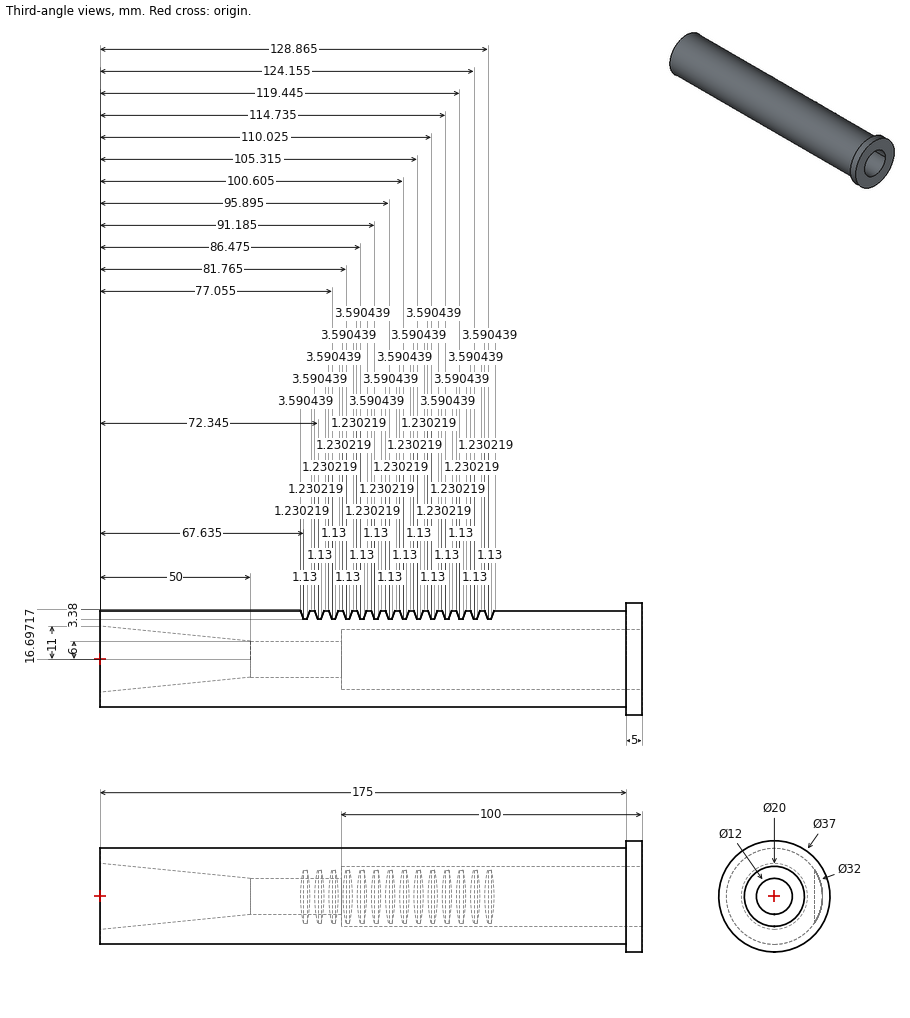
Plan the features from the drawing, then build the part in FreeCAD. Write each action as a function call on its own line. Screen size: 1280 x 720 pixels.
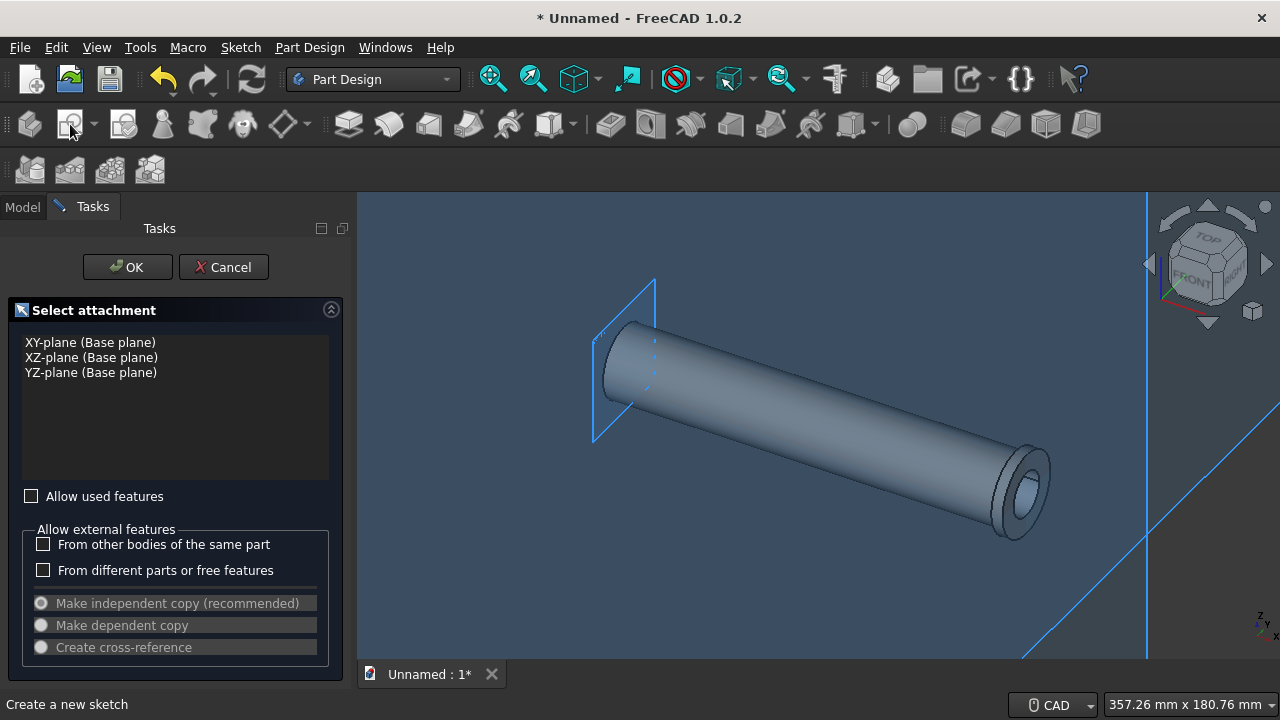
click(82, 342)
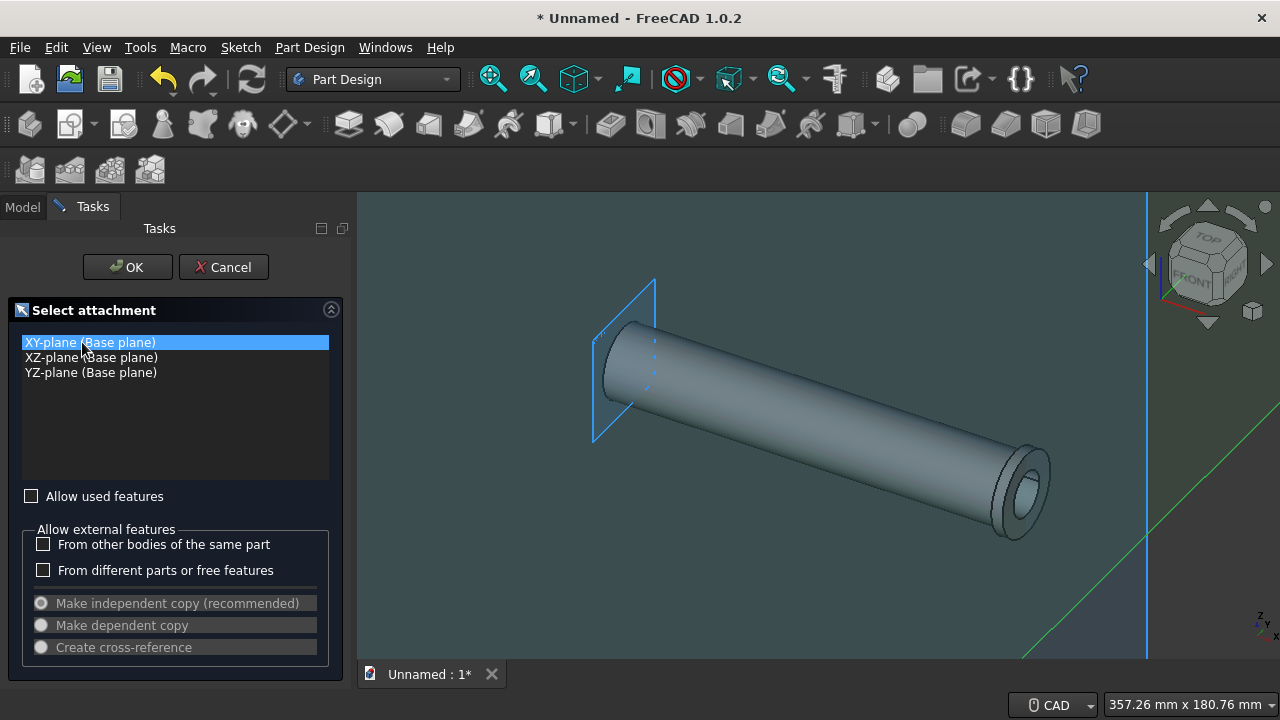
click(128, 267)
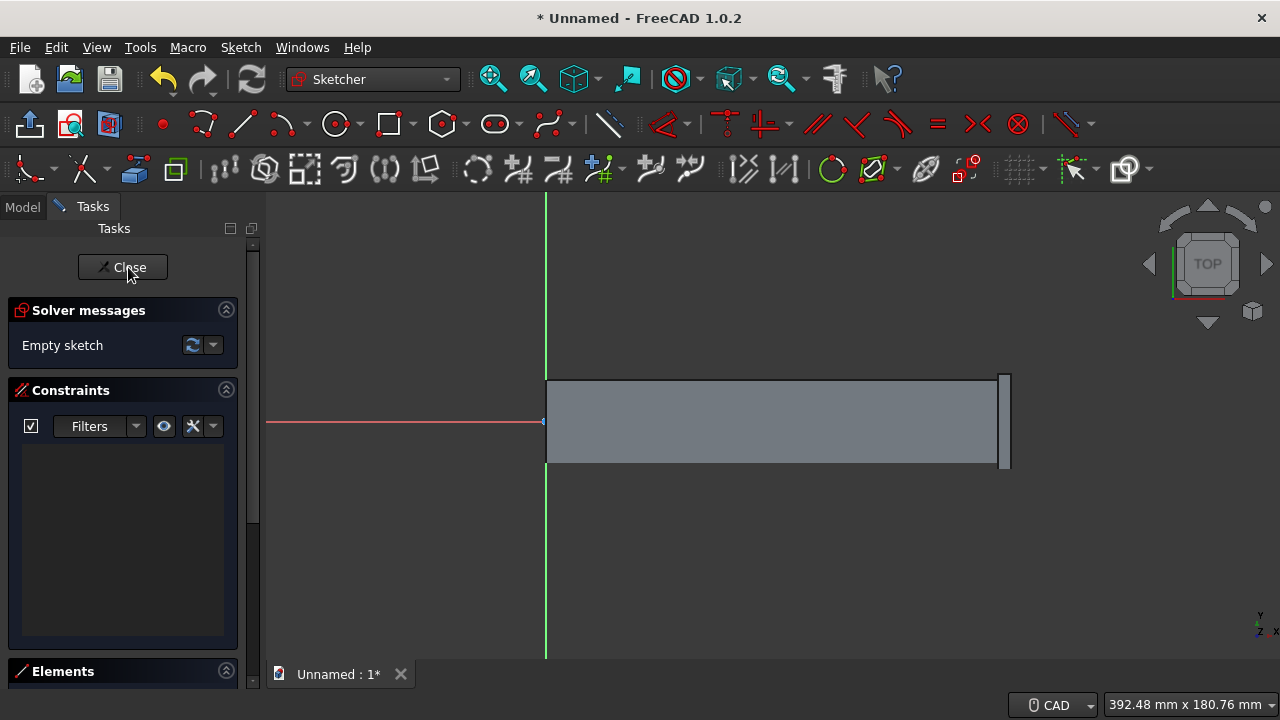
click(110, 124)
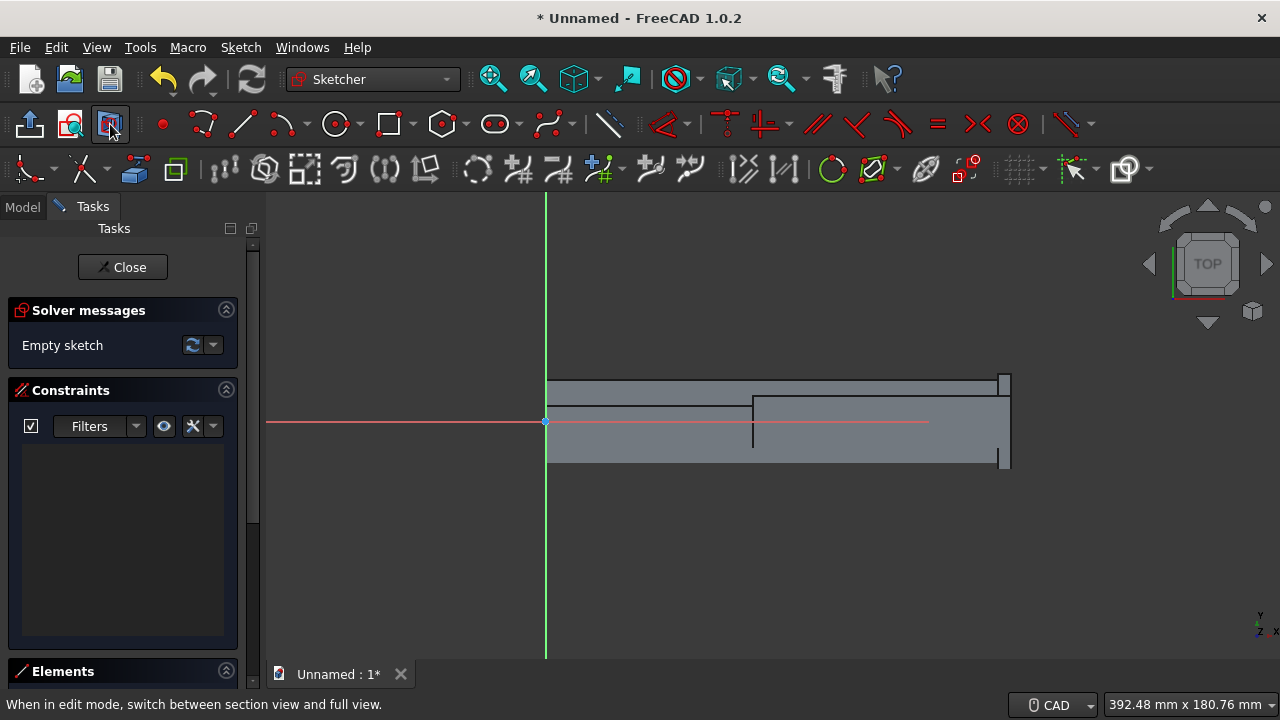
scroll(587, 403, up, 8)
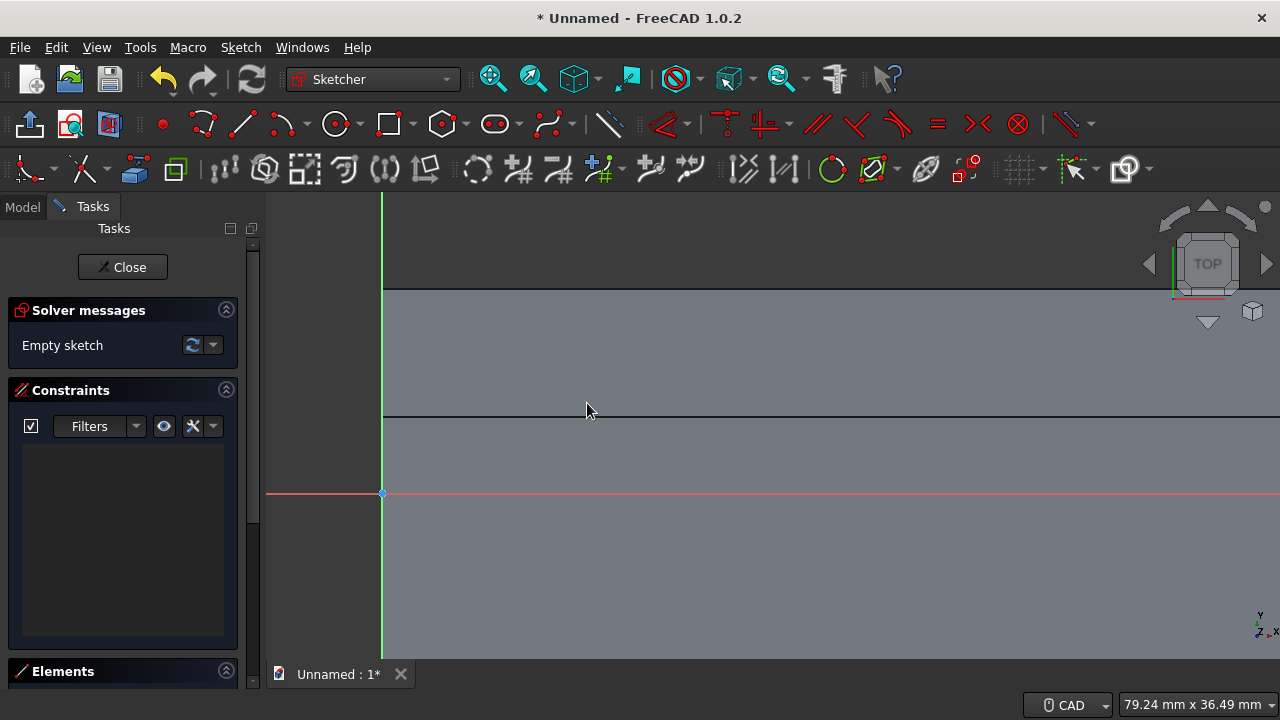
key(g)
key(m)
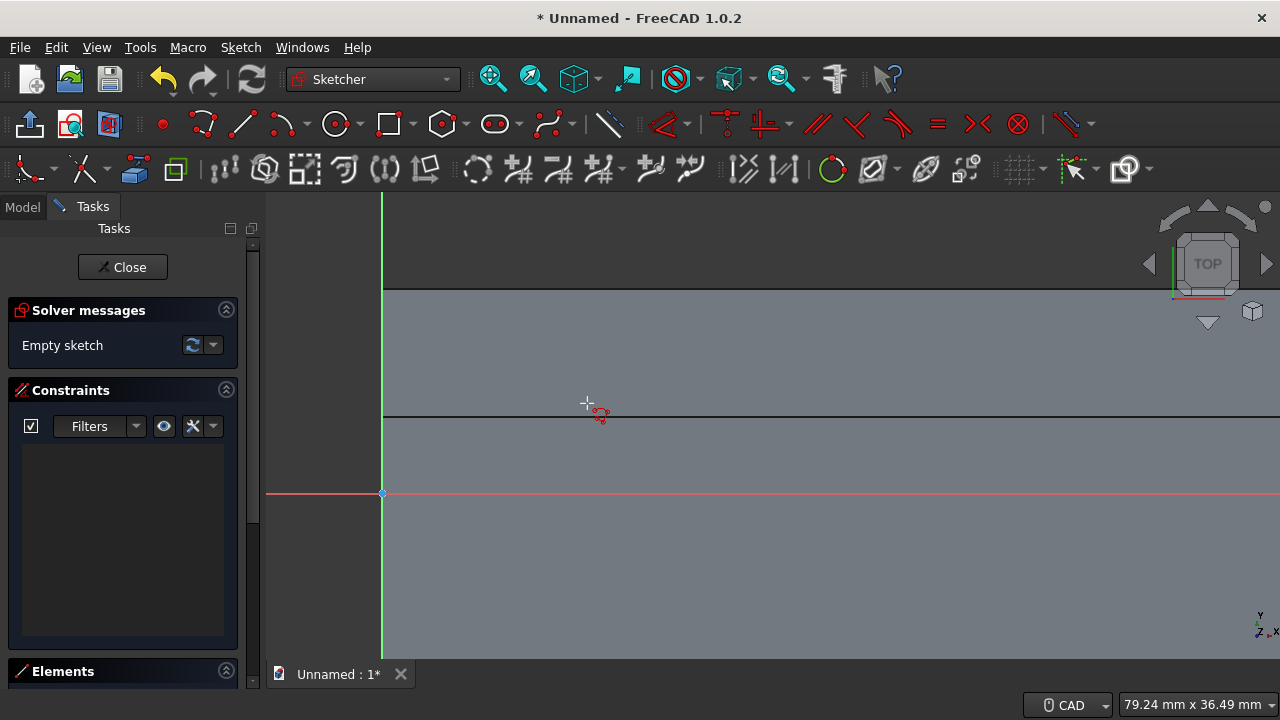
click(382, 494)
click(1022, 485)
click(1022, 417)
click(391, 353)
click(382, 494)
key(Escape)
key(Escape)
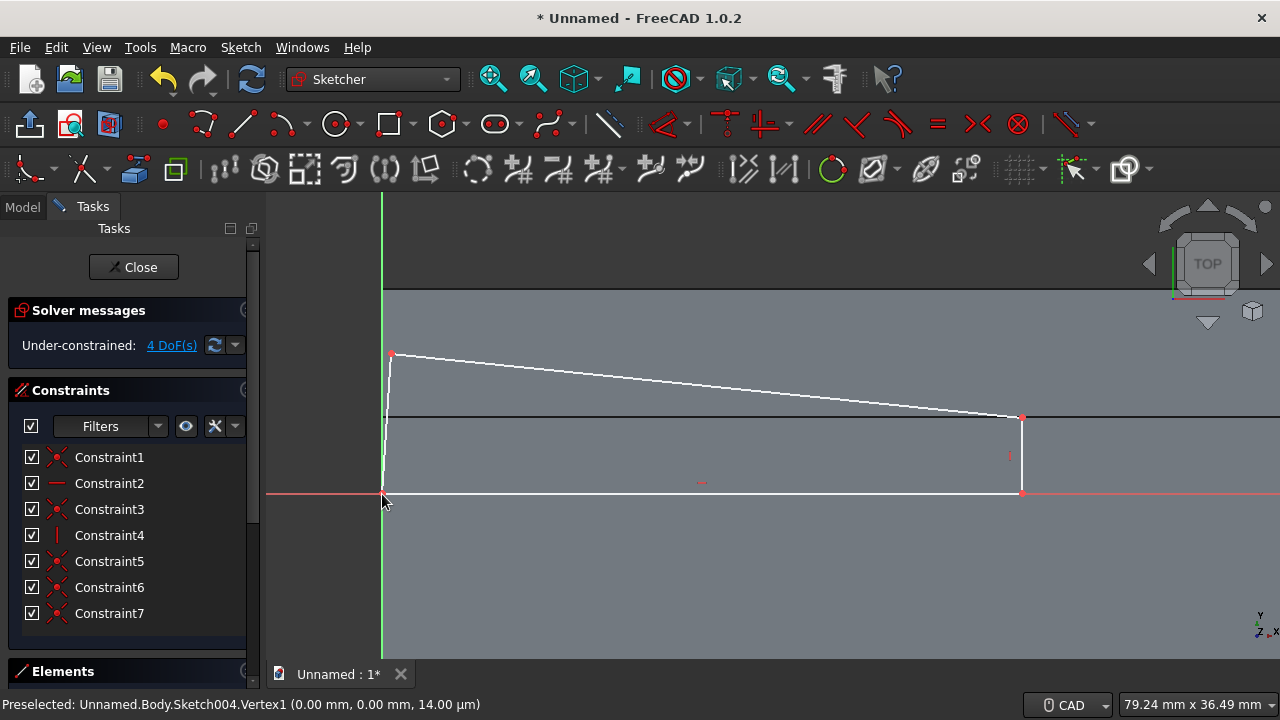
click(385, 452)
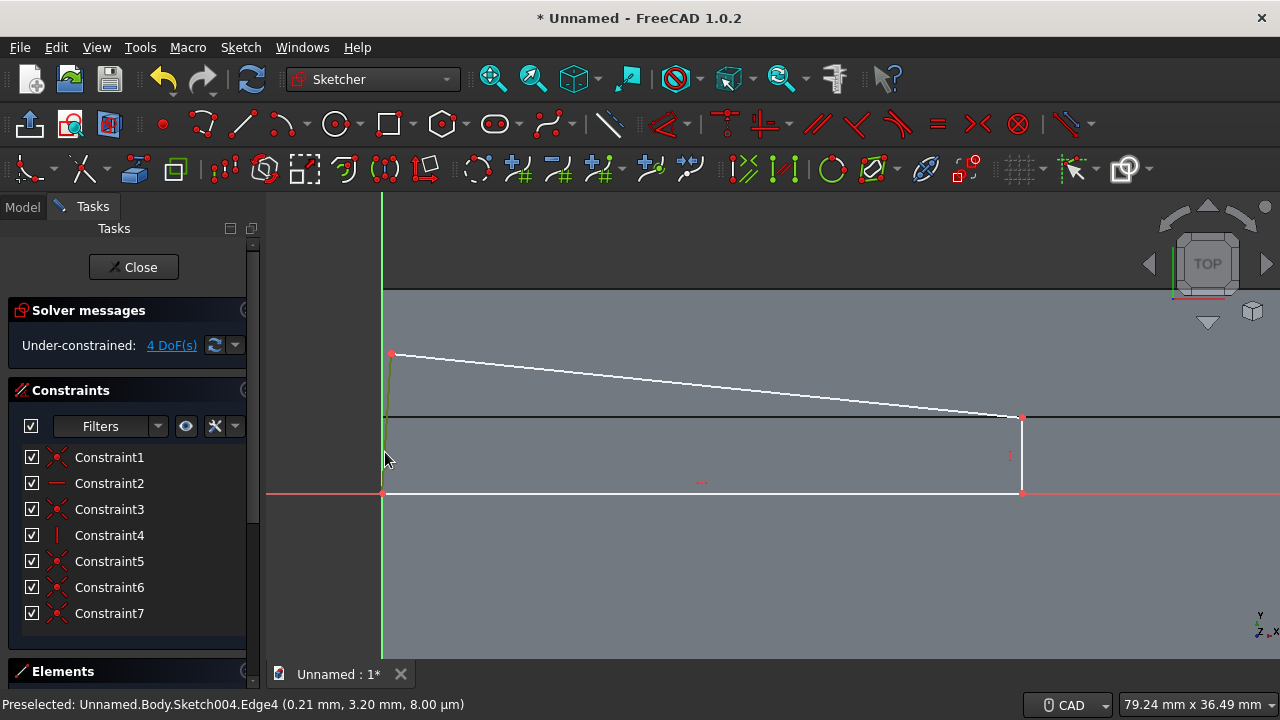
key(v)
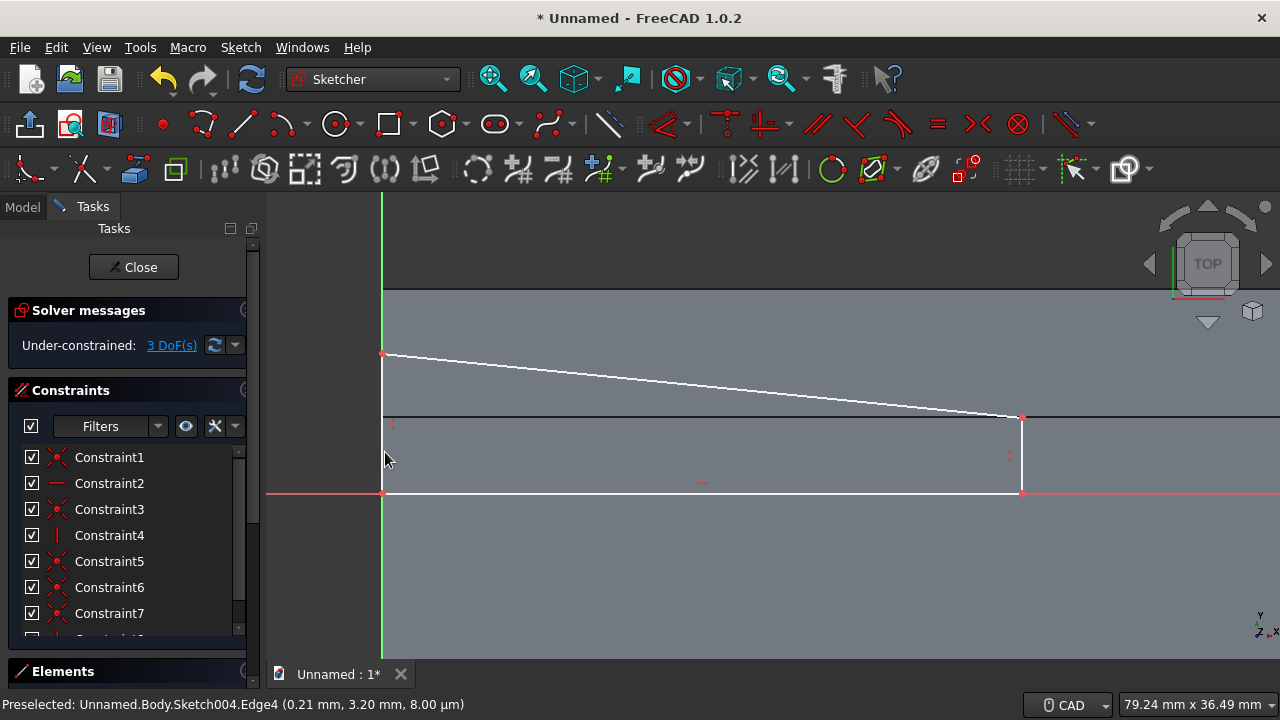
key(d)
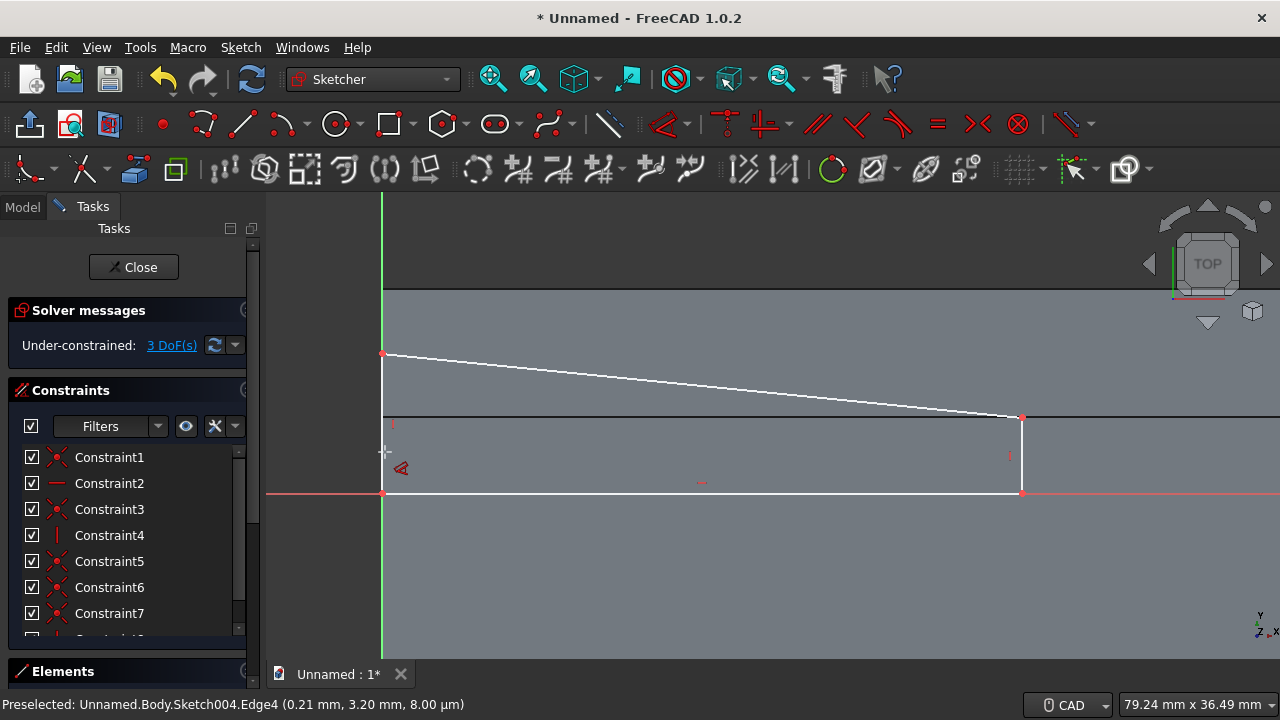
click(1022, 471)
click(1056, 456)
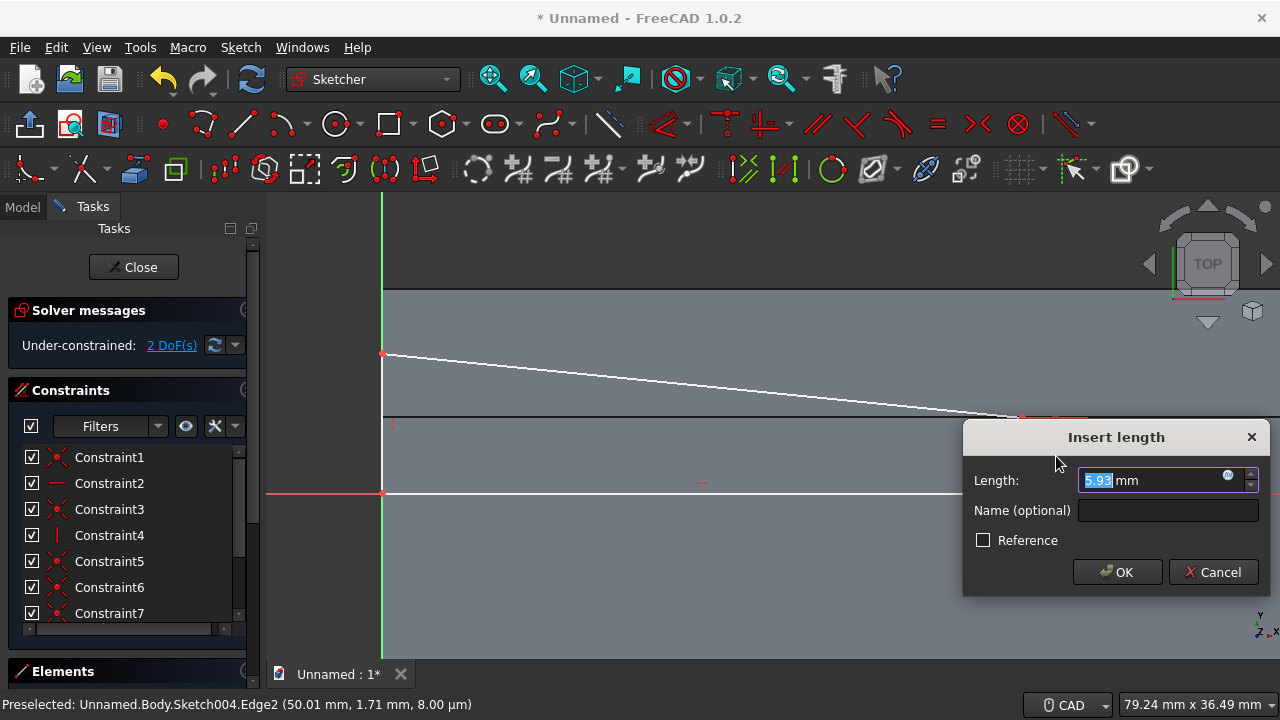
text(6)
key(Return)